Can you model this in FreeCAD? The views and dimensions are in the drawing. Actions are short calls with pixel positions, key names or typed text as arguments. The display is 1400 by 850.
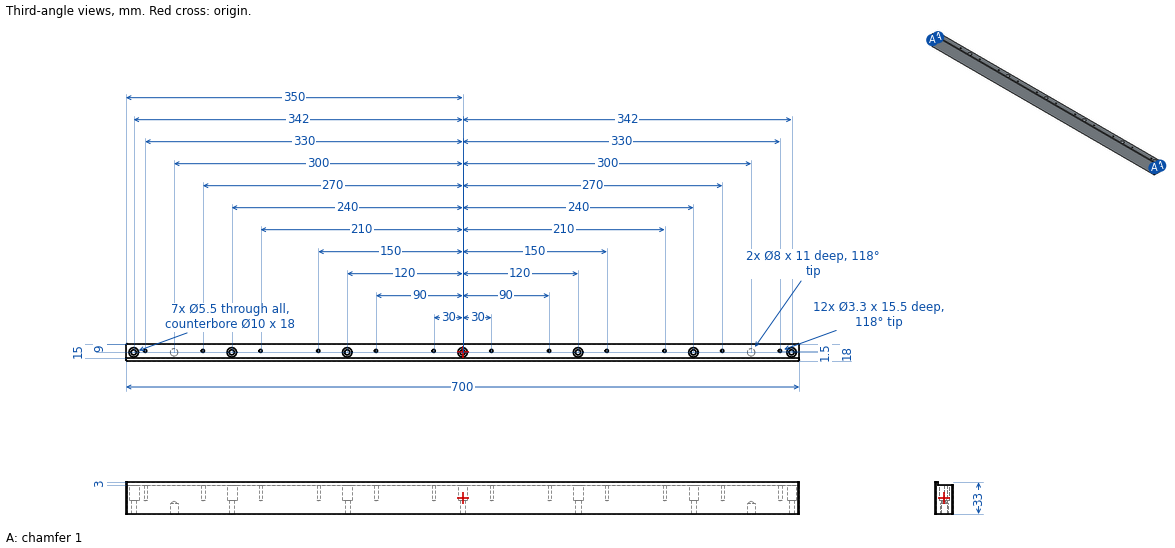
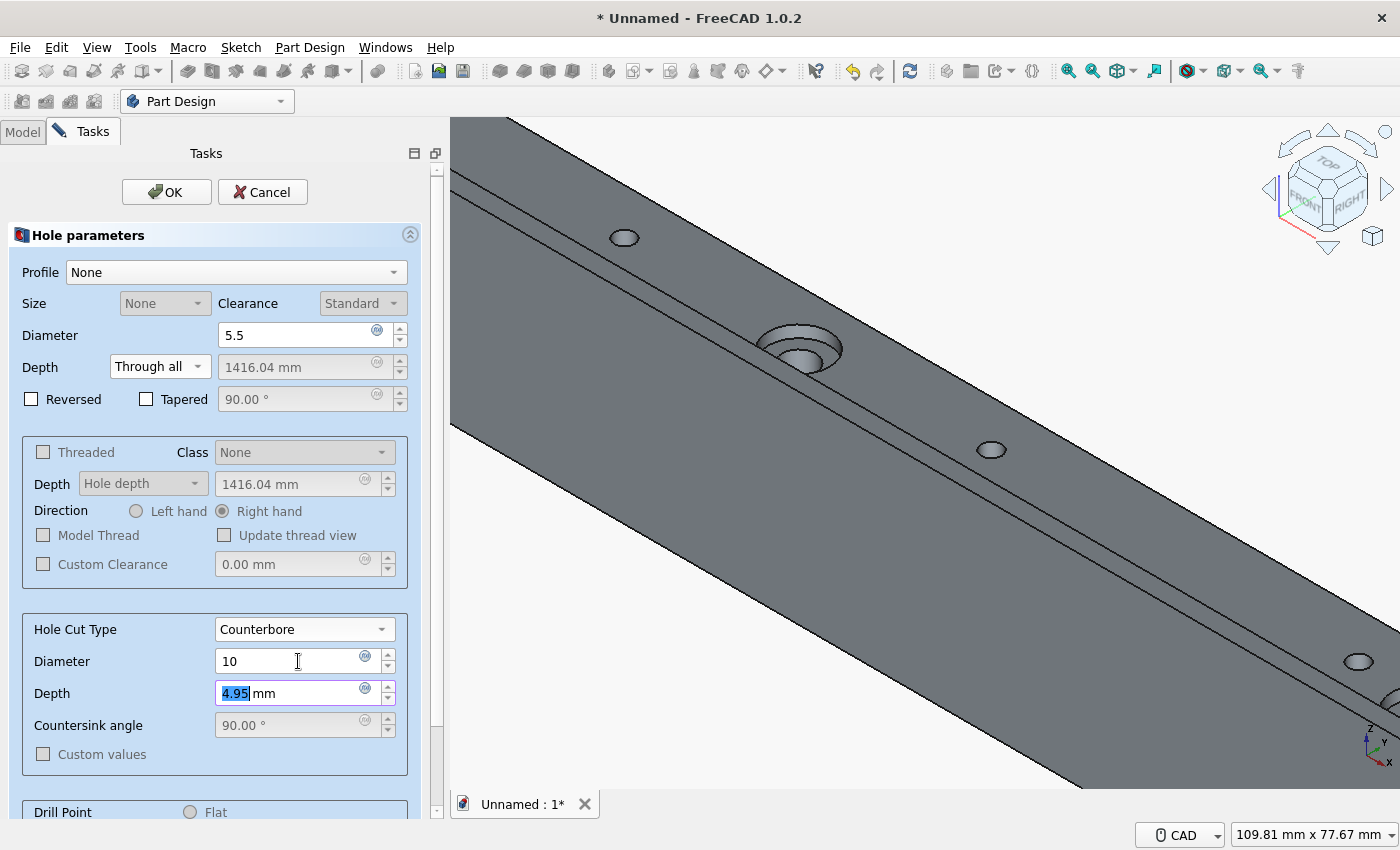
text(18)
key(Tab)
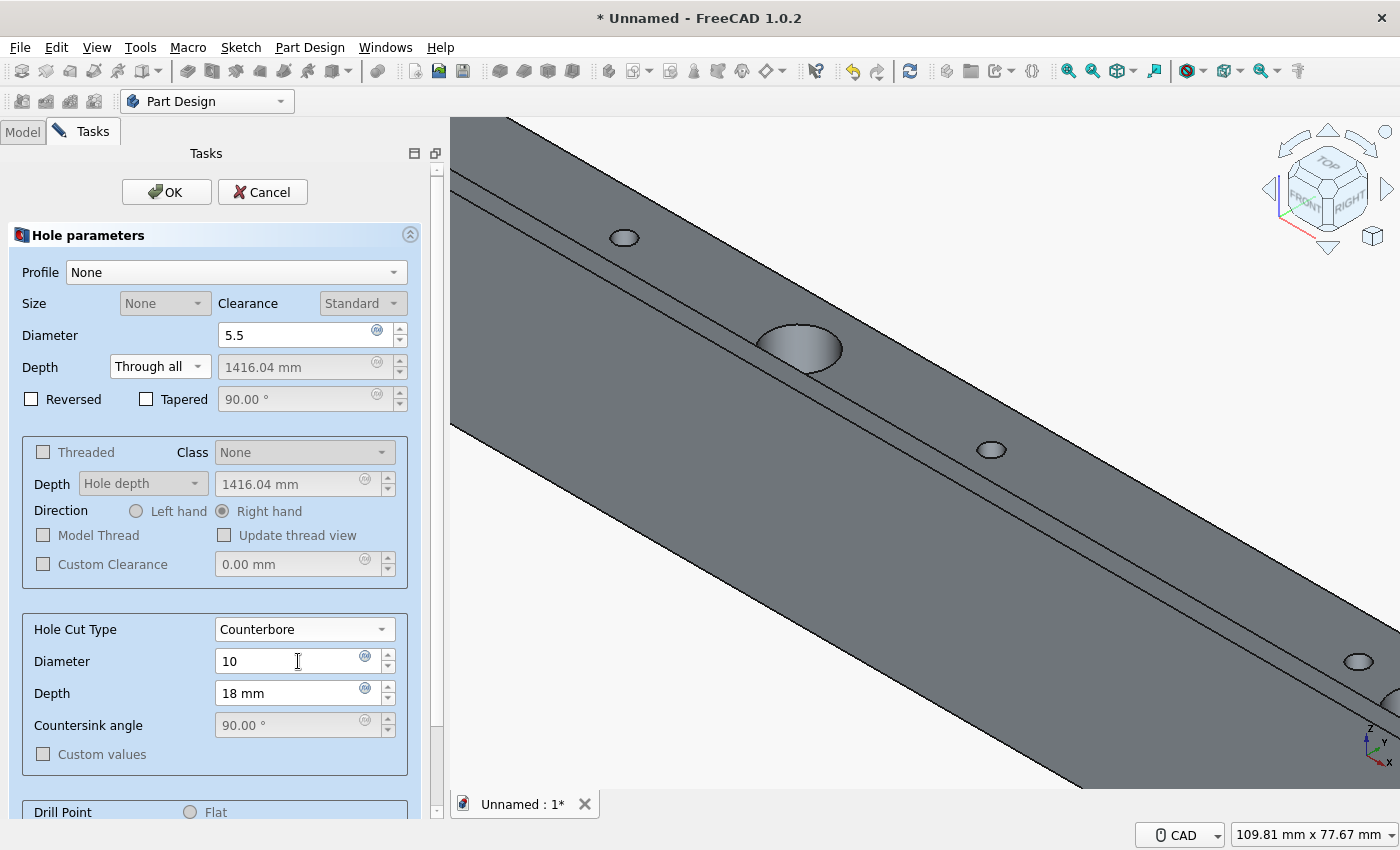
click(167, 192)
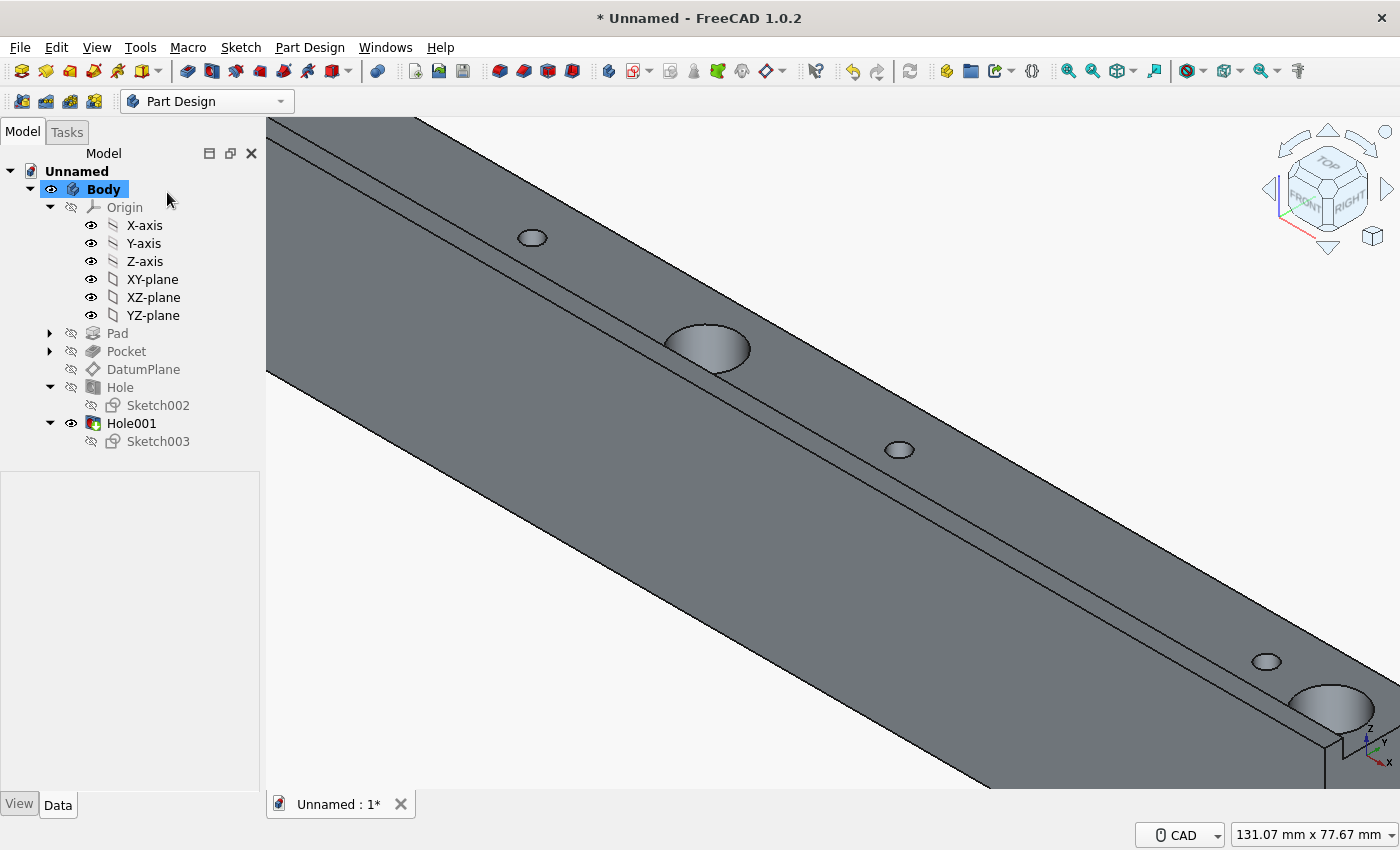
click(1070, 72)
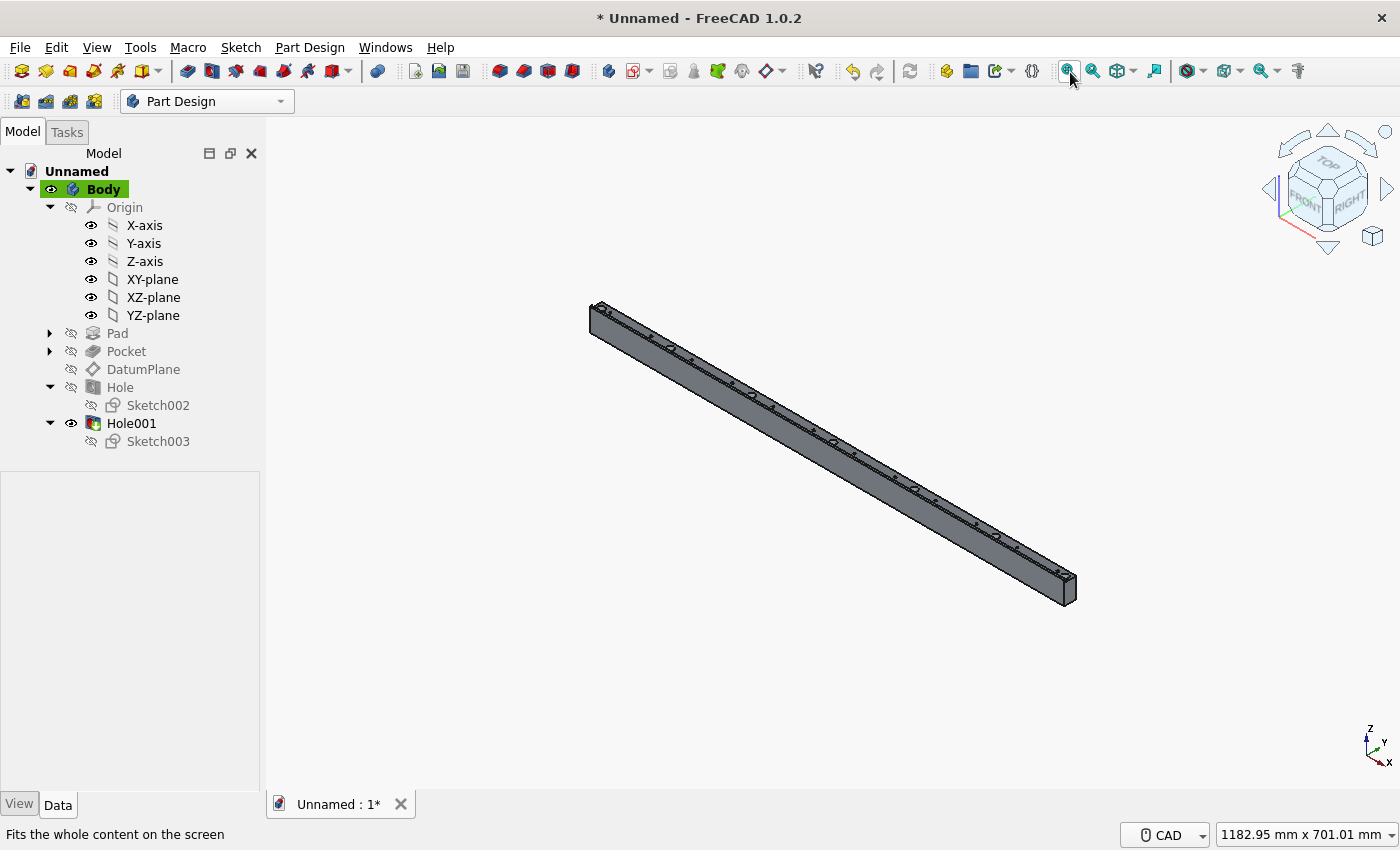
key(5)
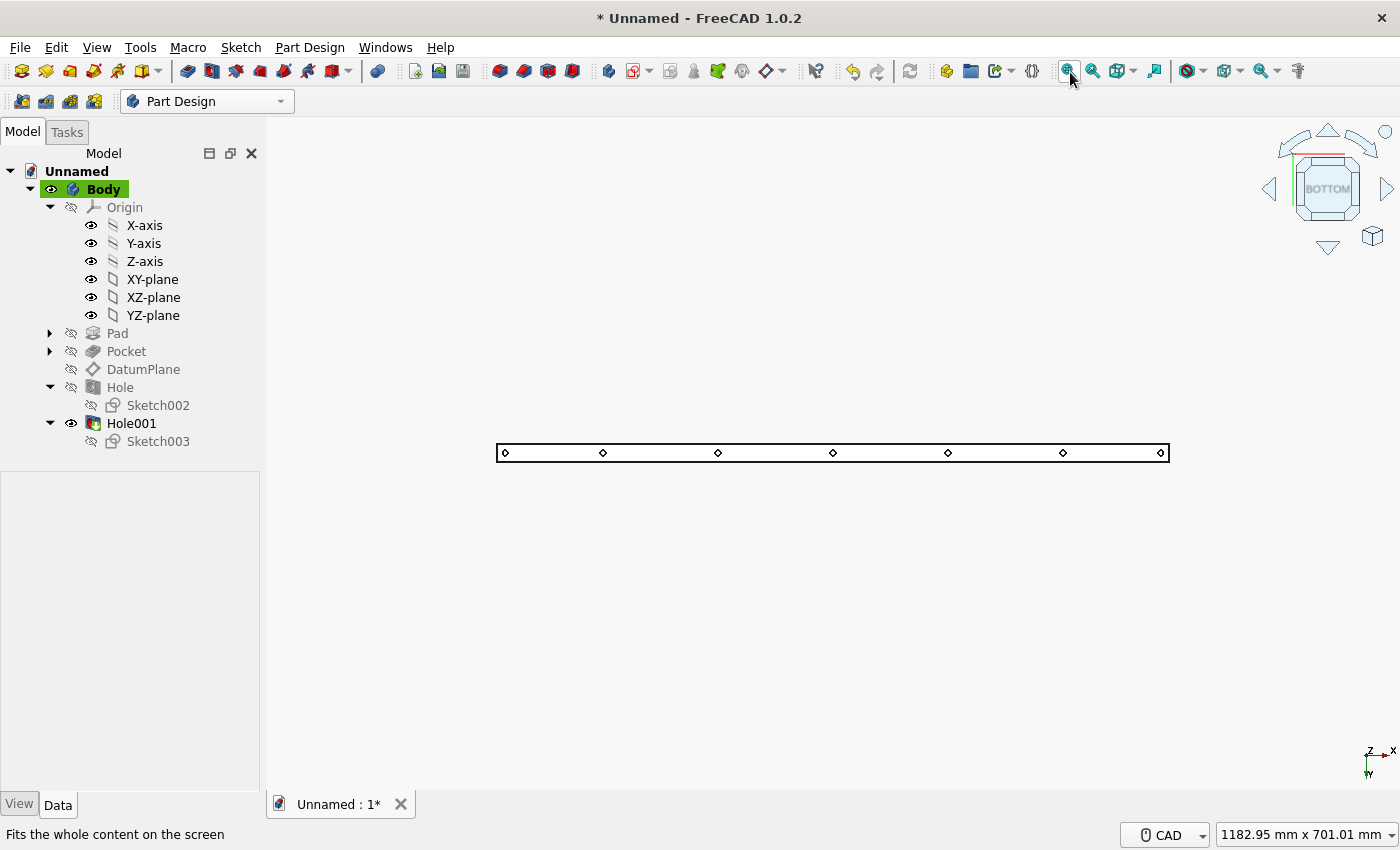
click(1121, 452)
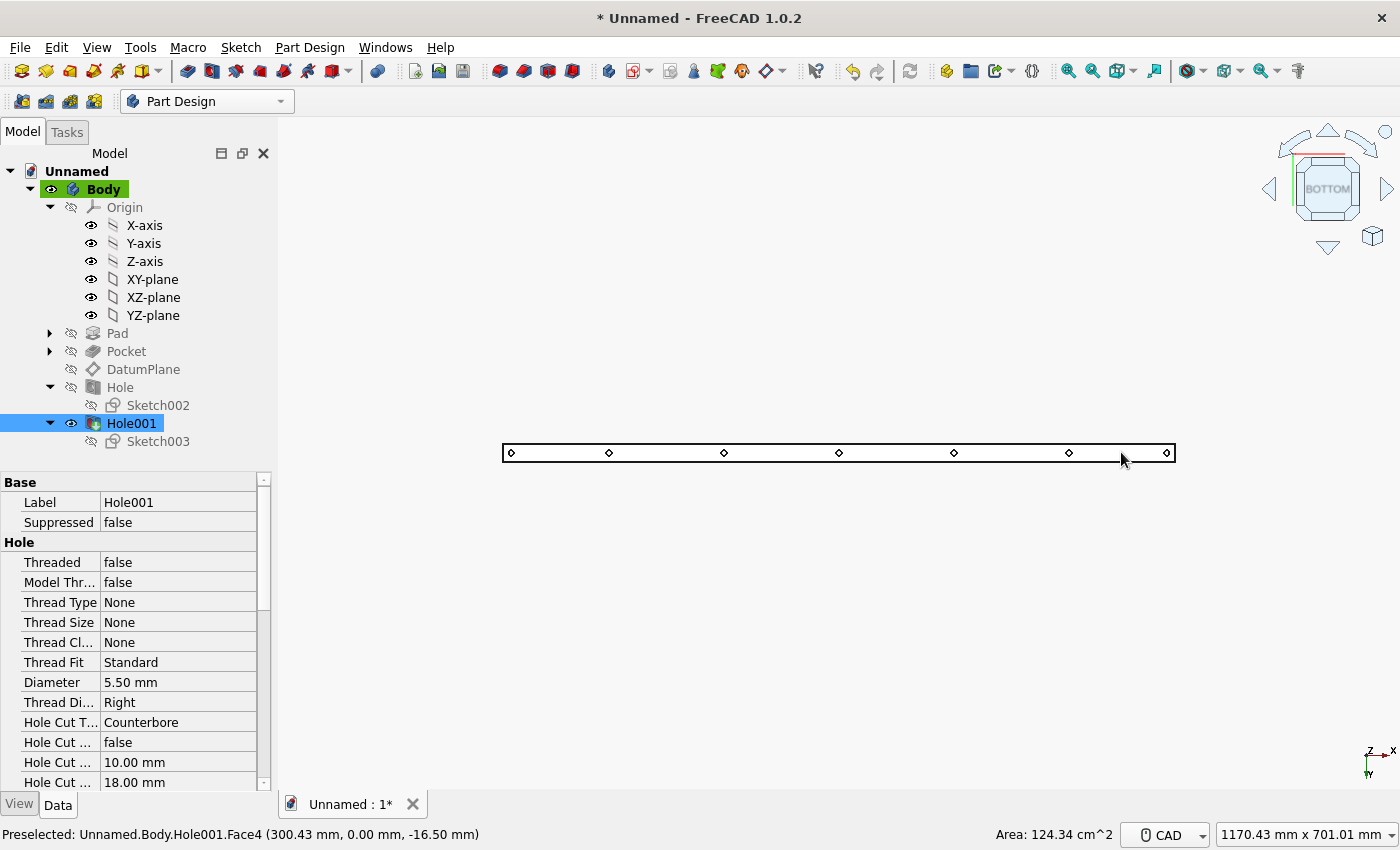
click(634, 72)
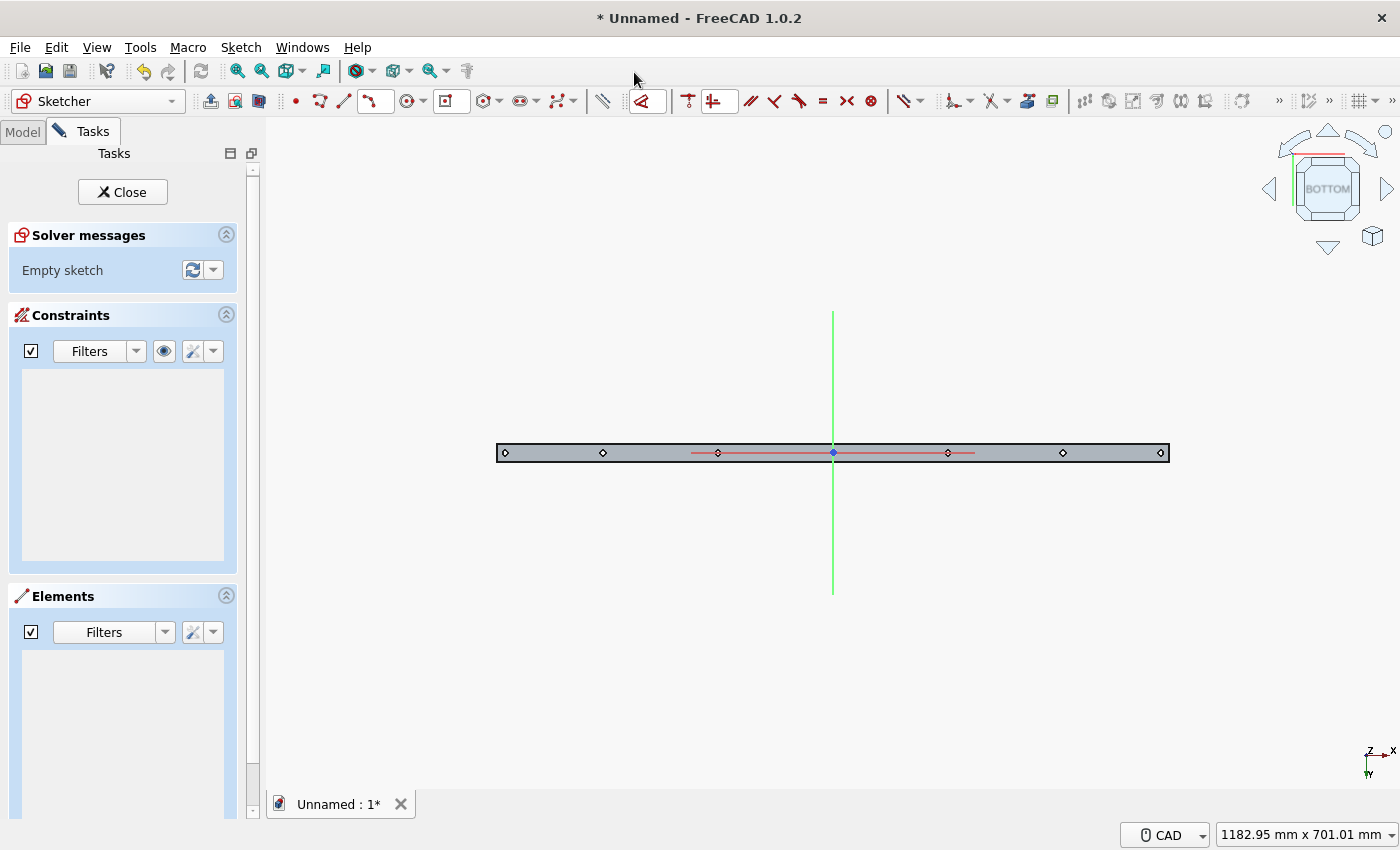
click(408, 102)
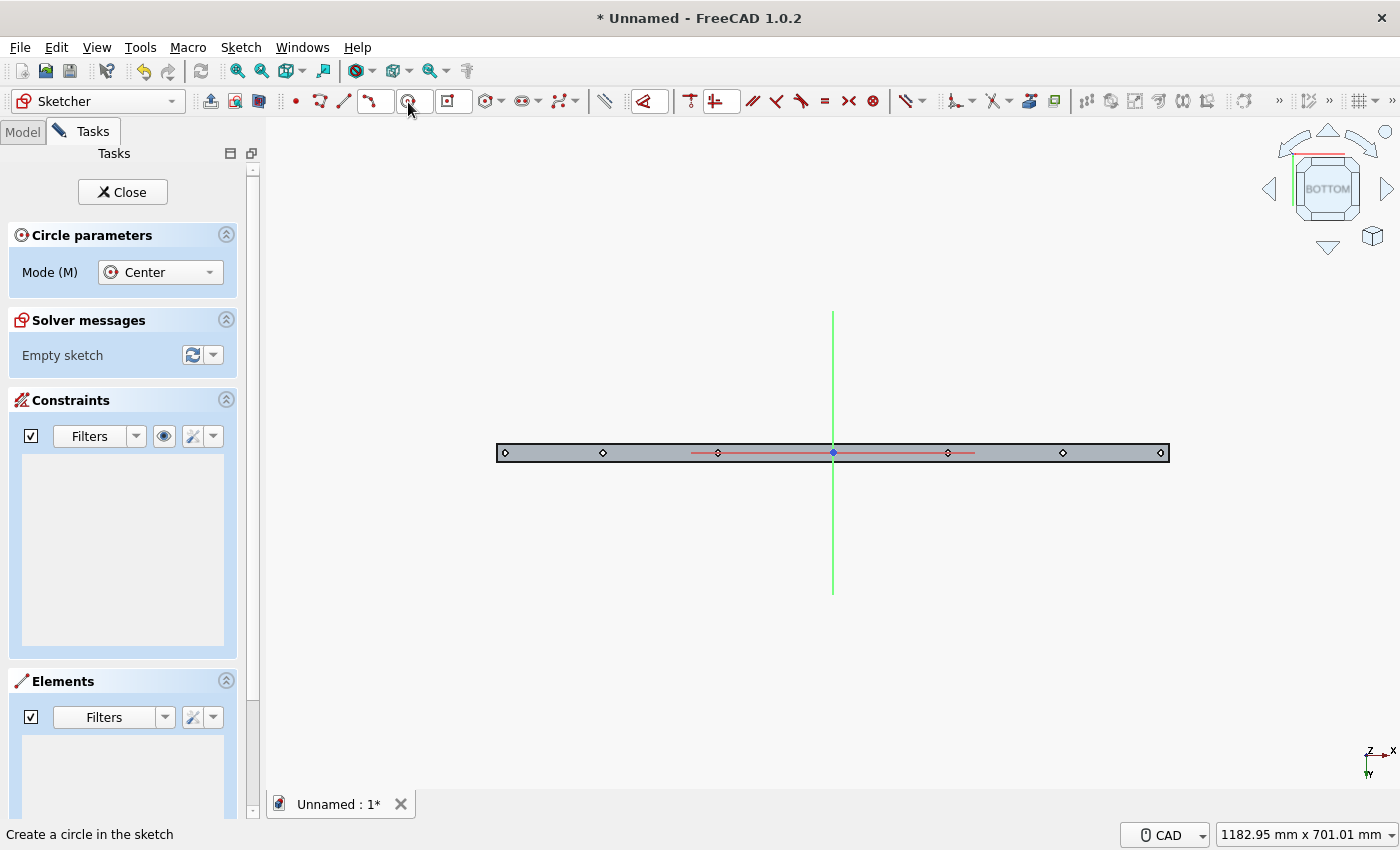
scroll(1121, 453, up, 9)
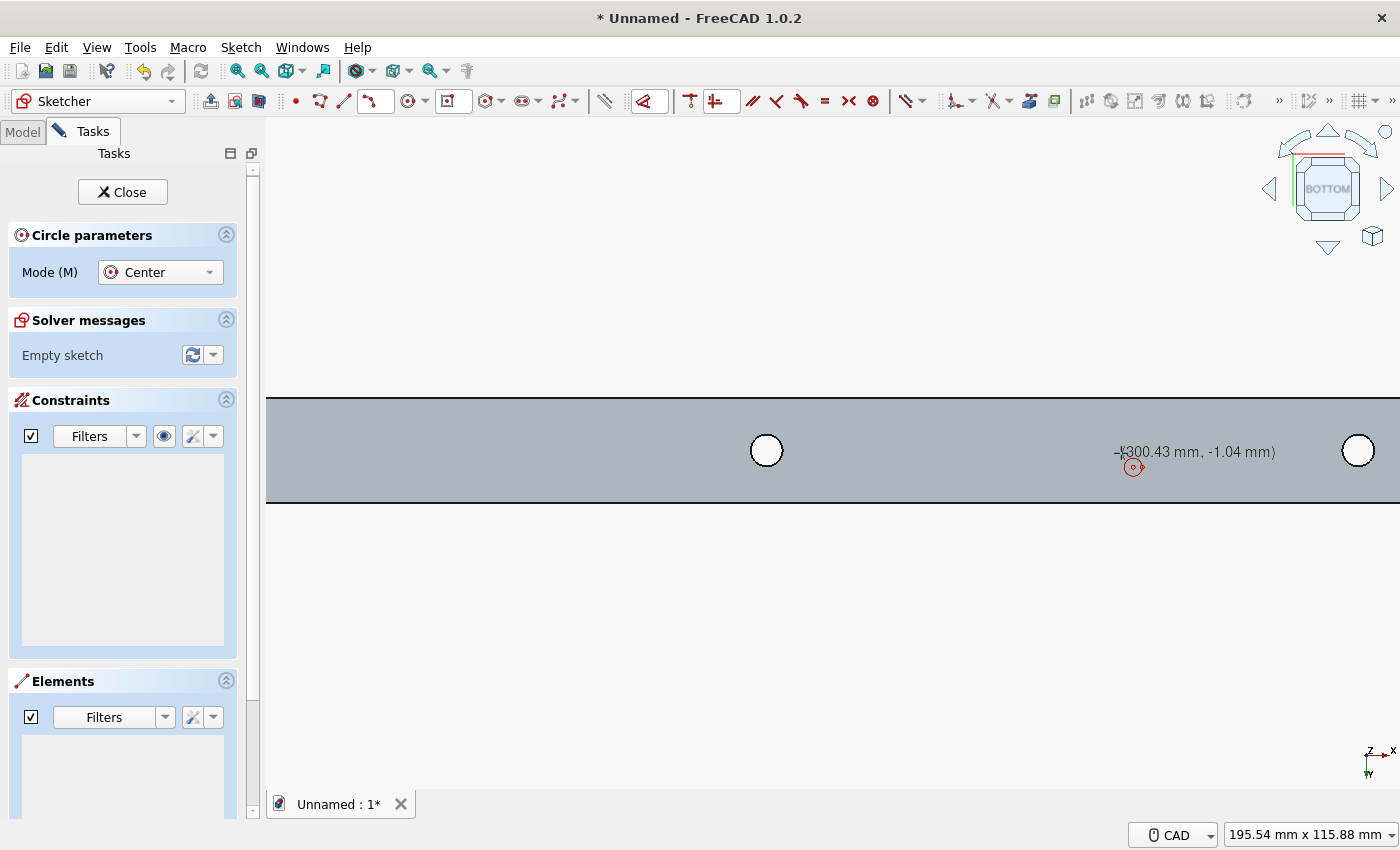
scroll(1116, 454, down, 8)